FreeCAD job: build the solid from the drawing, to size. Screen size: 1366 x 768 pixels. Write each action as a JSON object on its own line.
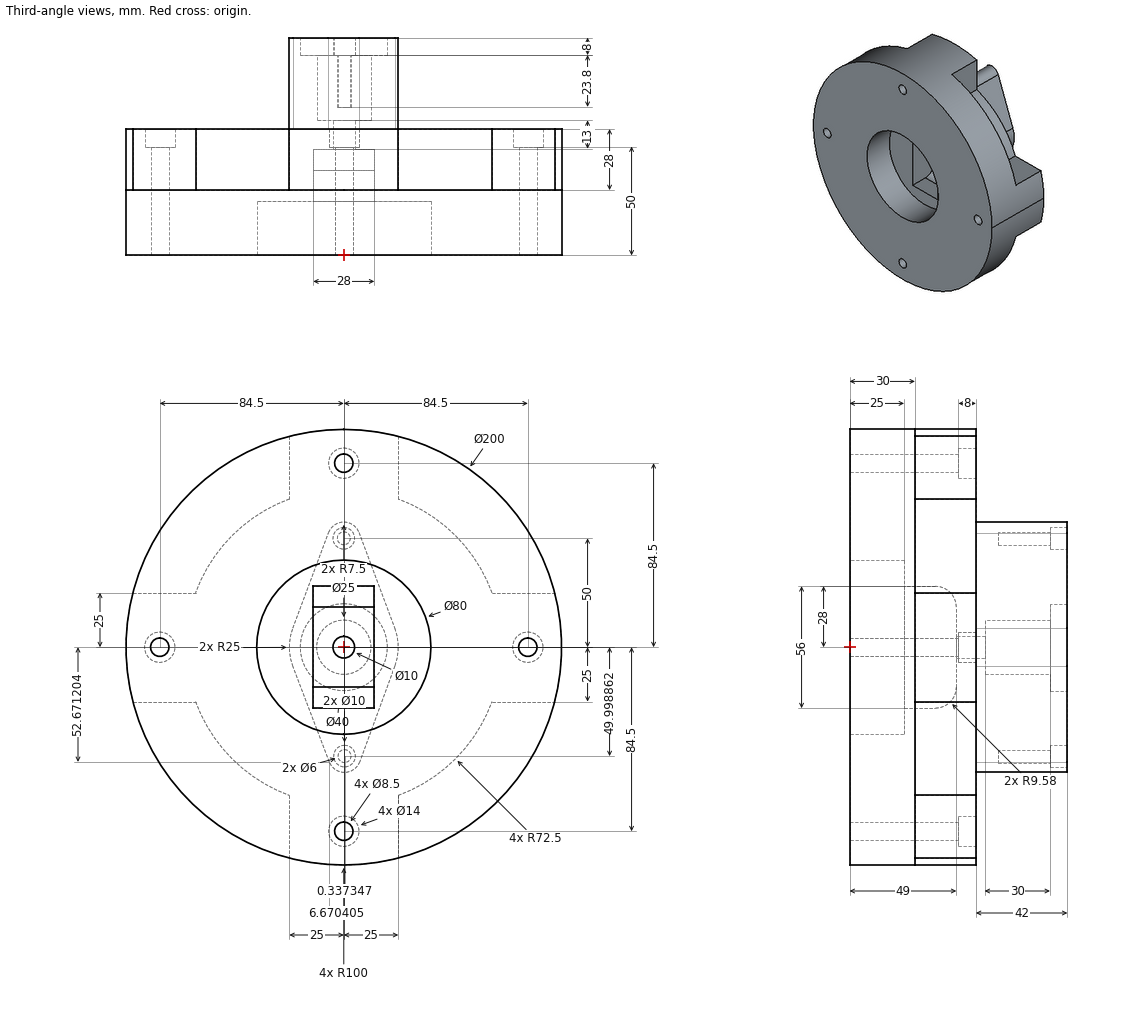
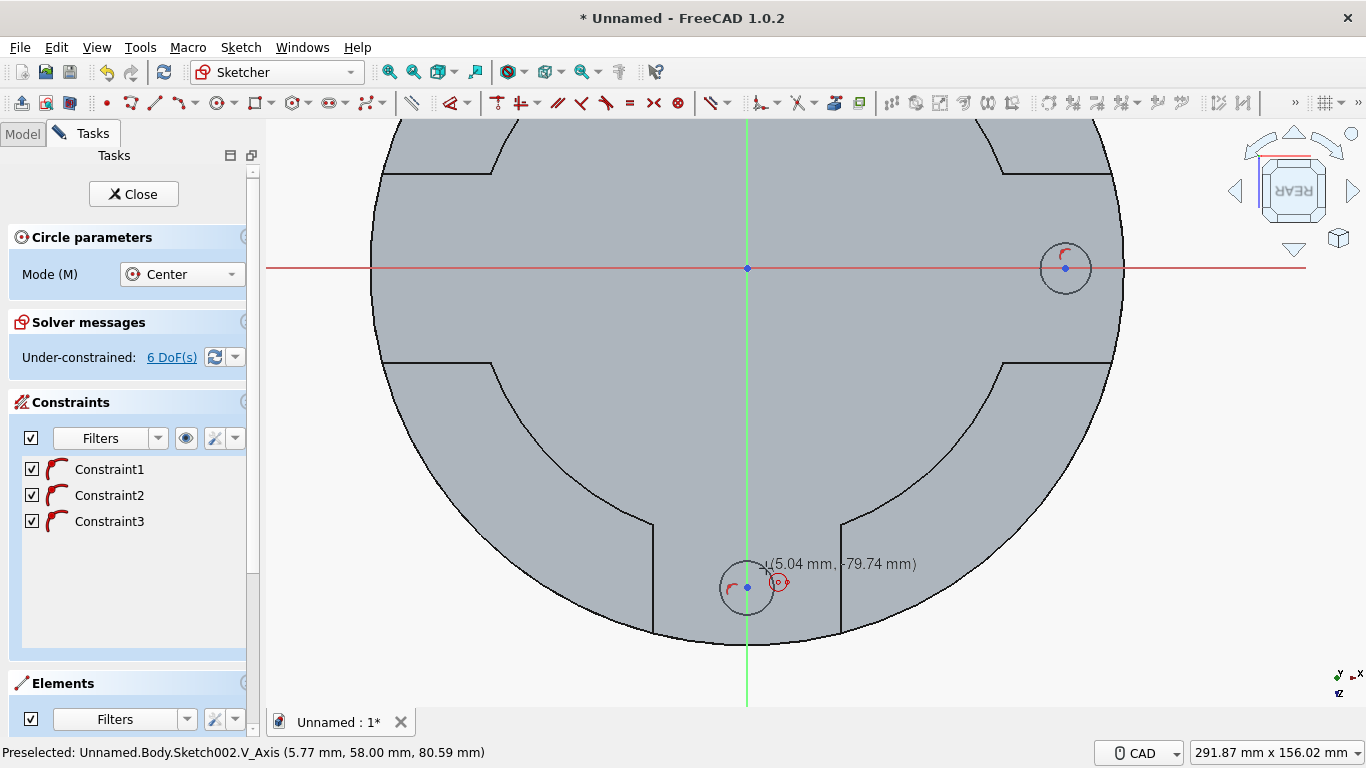
{"action": "left_click", "coordinate": [429, 268]}
{"action": "left_click", "coordinate": [447, 250]}
{"action": "key", "text": "Escape"}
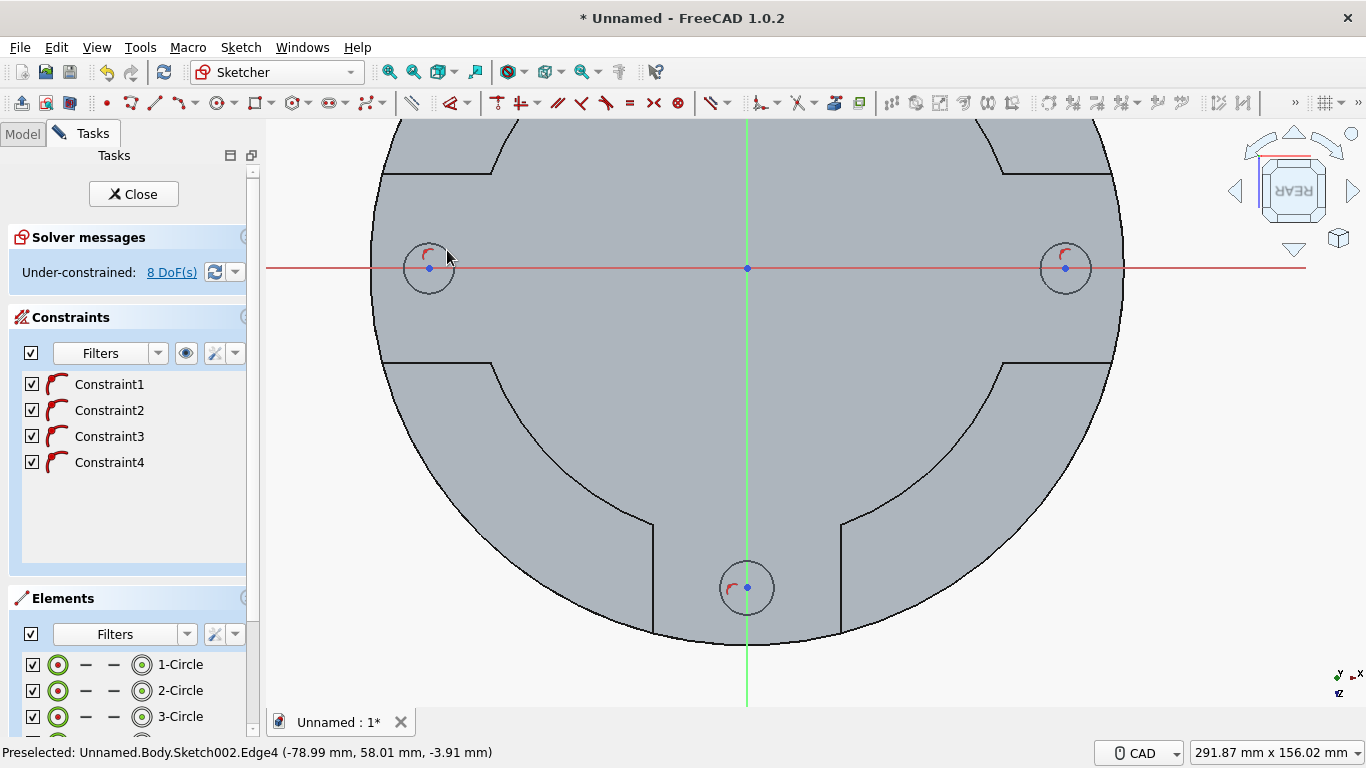
{"action": "scroll", "coordinate": [748, 589], "scroll_direction": "down", "scroll_amount": 3}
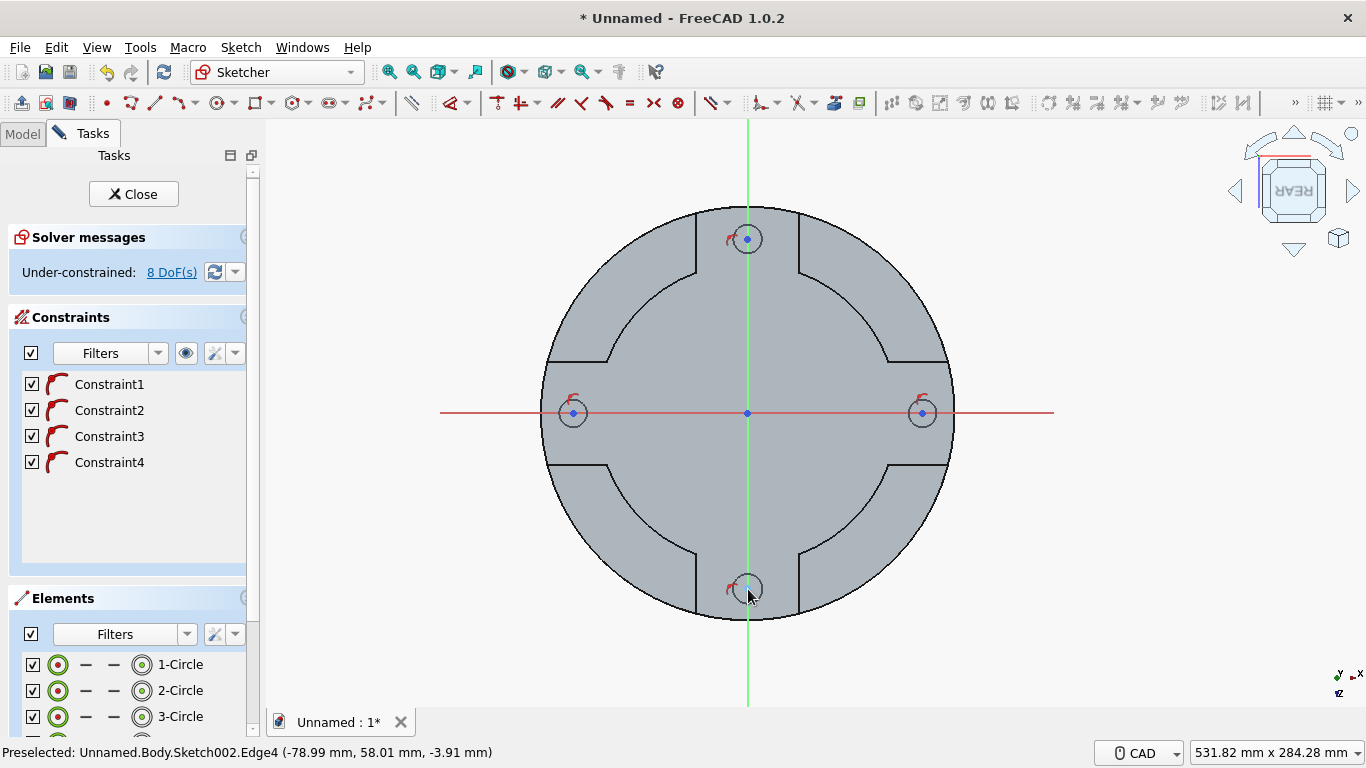
{"action": "scroll", "coordinate": [758, 229], "scroll_direction": "up", "scroll_amount": 2}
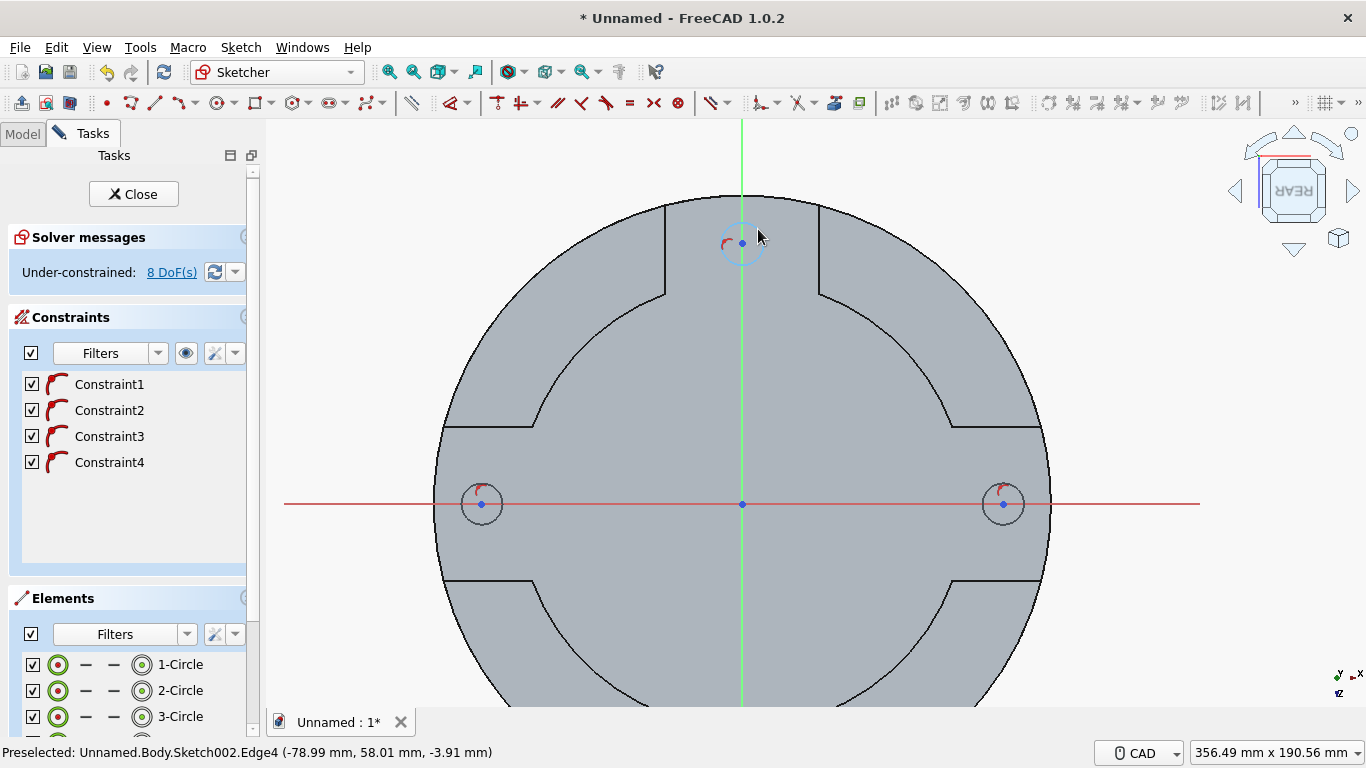
{"action": "left_click", "coordinate": [757, 229]}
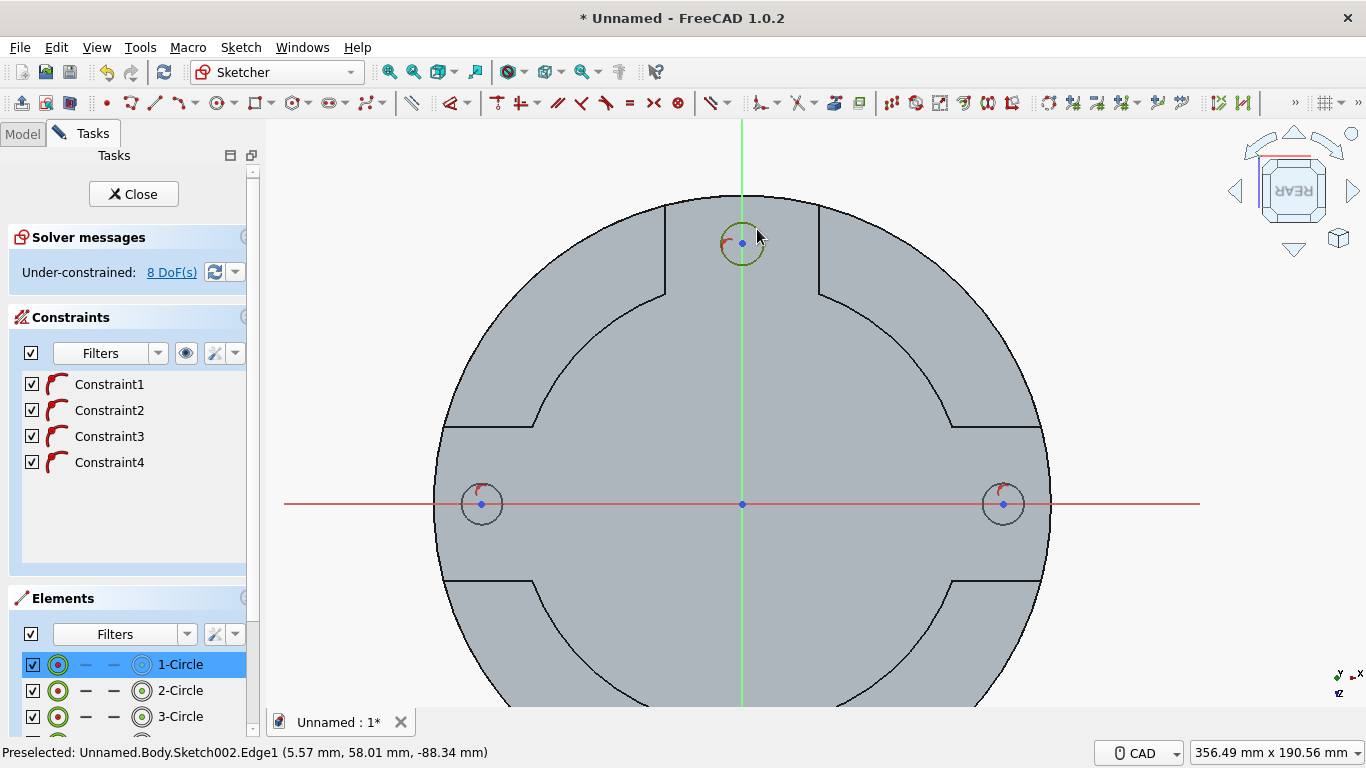
{"action": "left_click", "coordinate": [1018, 489]}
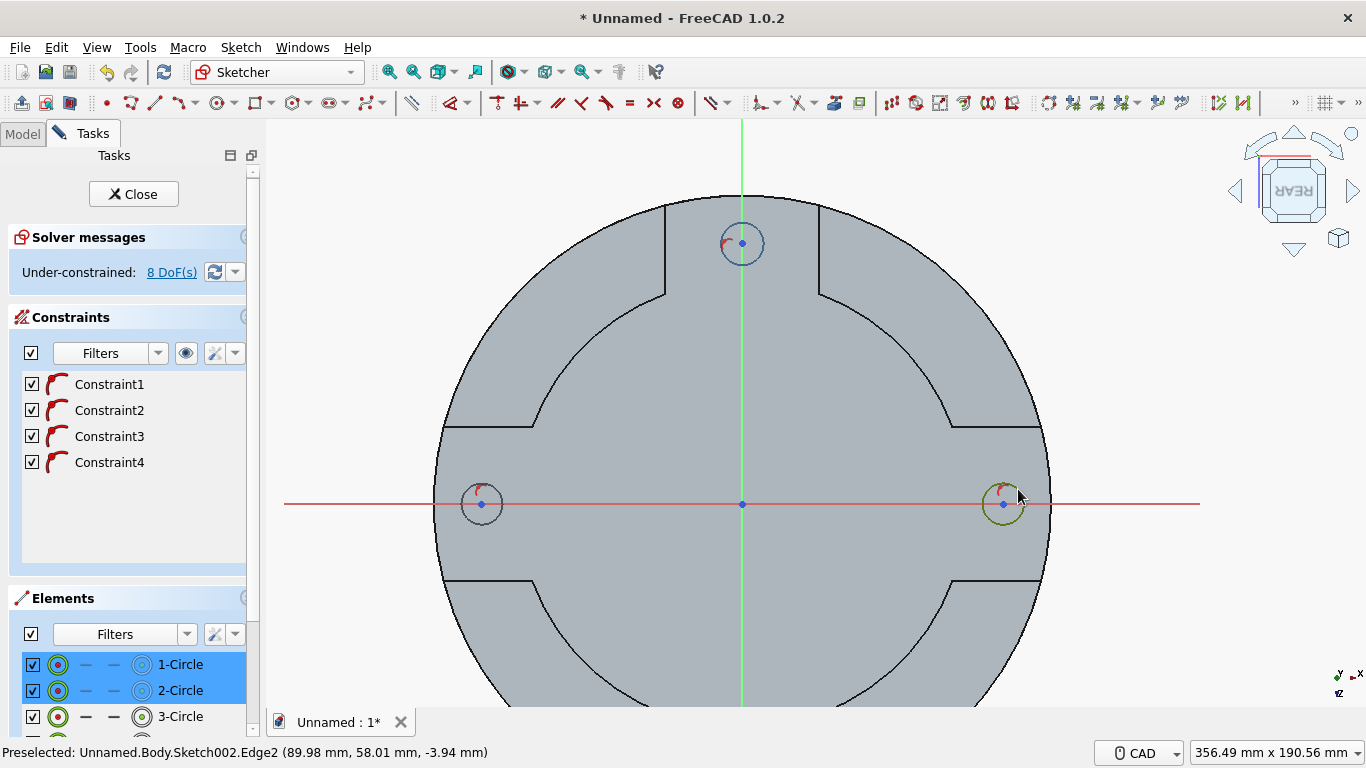
{"action": "scroll", "coordinate": [758, 228], "scroll_direction": "down", "scroll_amount": 2}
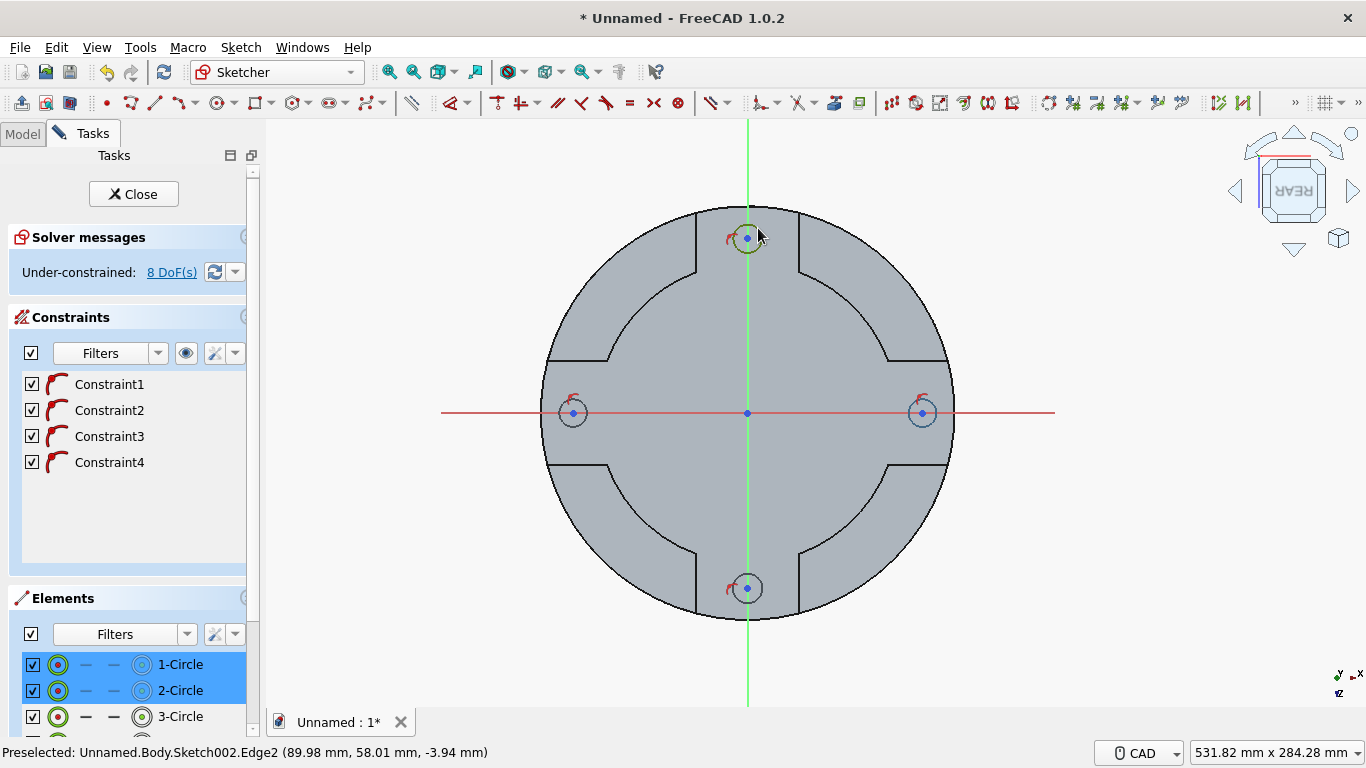
{"action": "scroll", "coordinate": [758, 578], "scroll_direction": "up", "scroll_amount": 2}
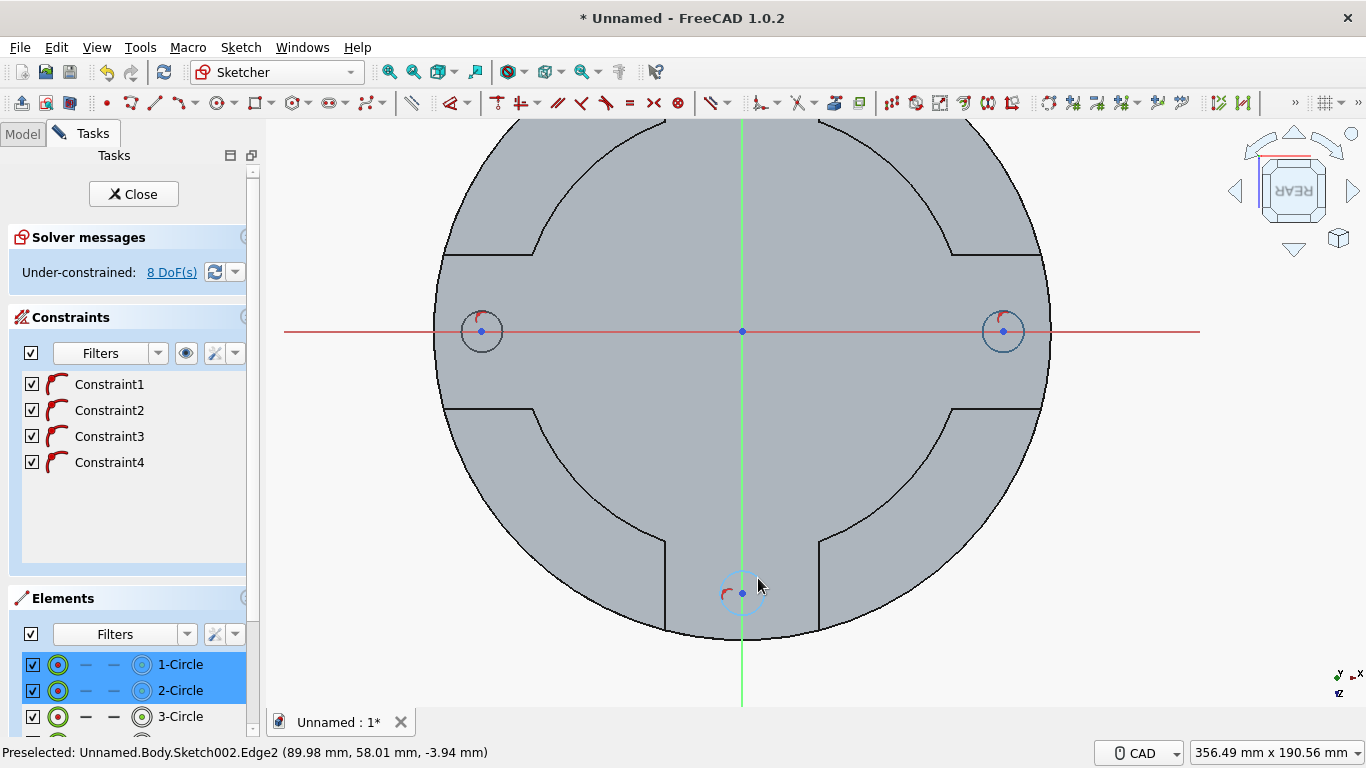
{"action": "left_click", "coordinate": [758, 578]}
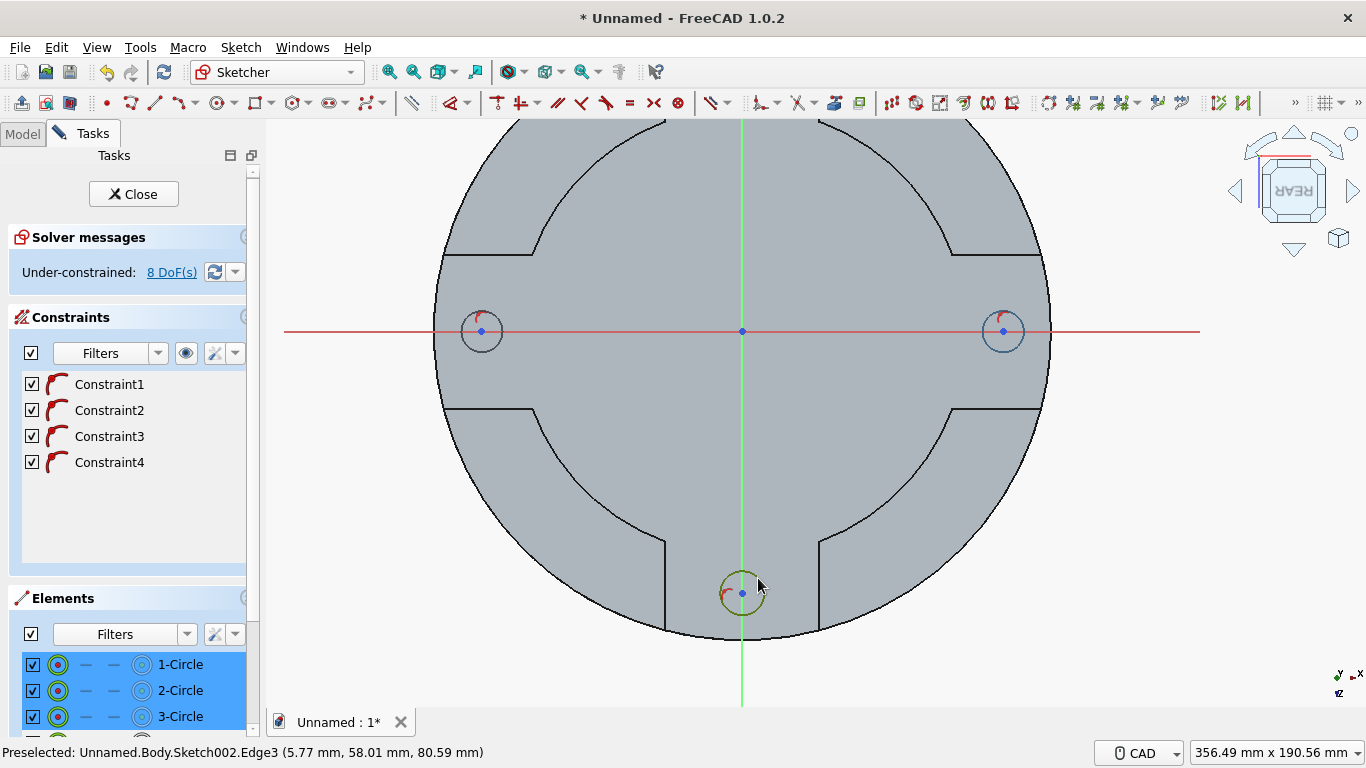
{"action": "left_click", "coordinate": [496, 317]}